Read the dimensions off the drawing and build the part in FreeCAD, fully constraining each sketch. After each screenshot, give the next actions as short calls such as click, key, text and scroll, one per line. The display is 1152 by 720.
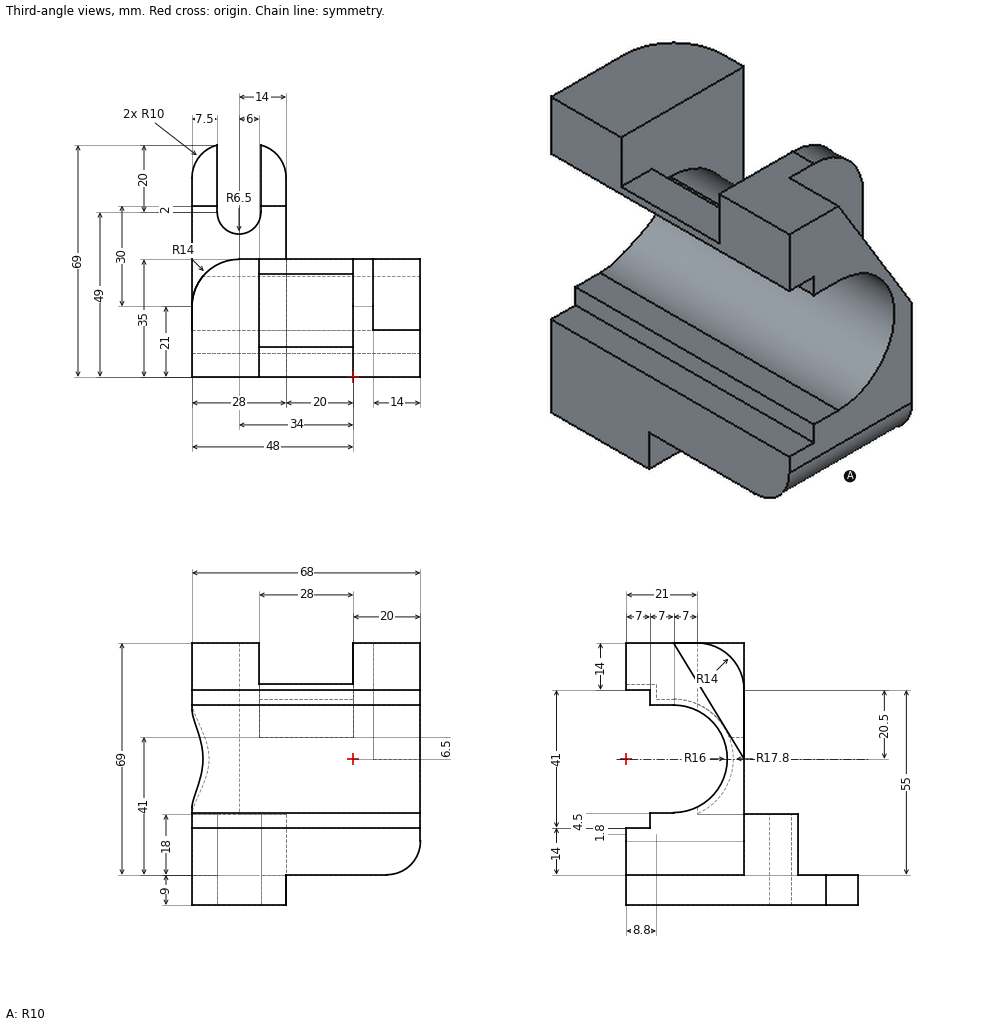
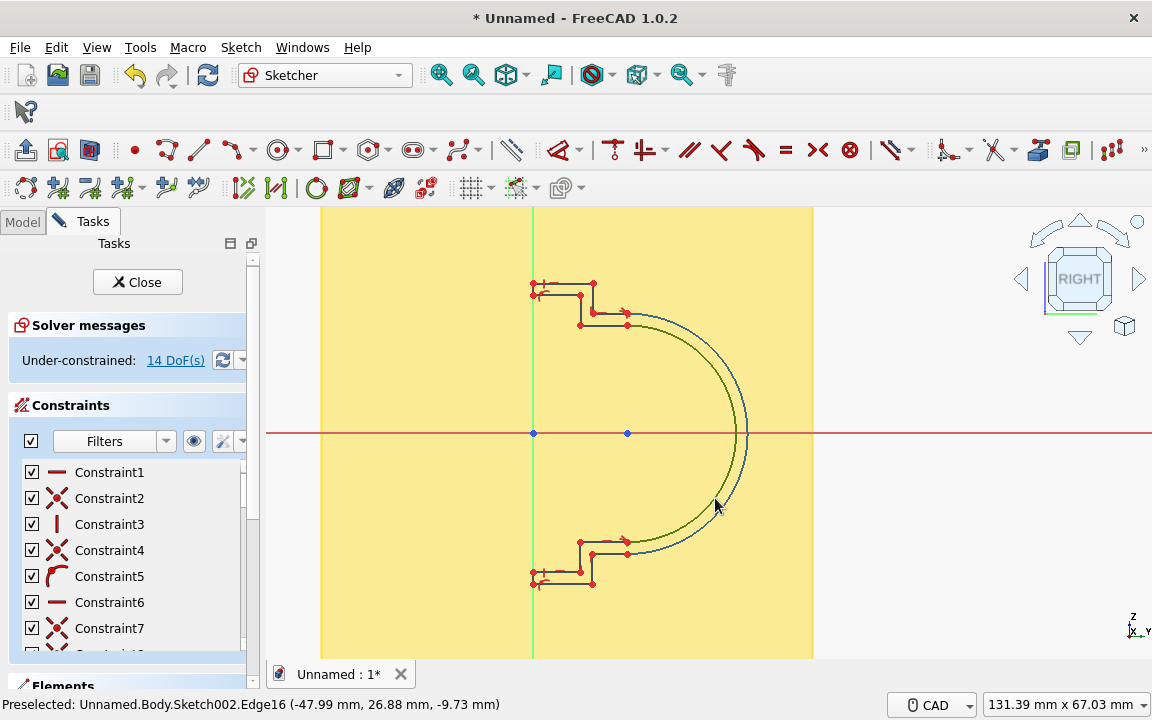
click(614, 150)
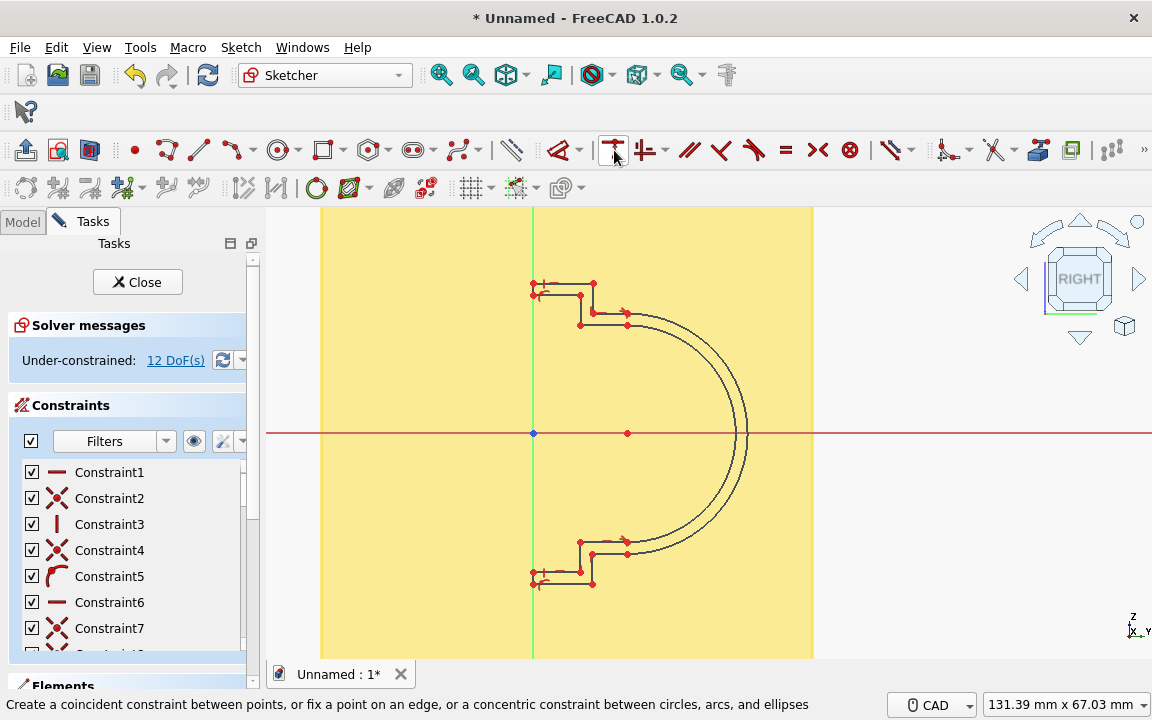
click(627, 434)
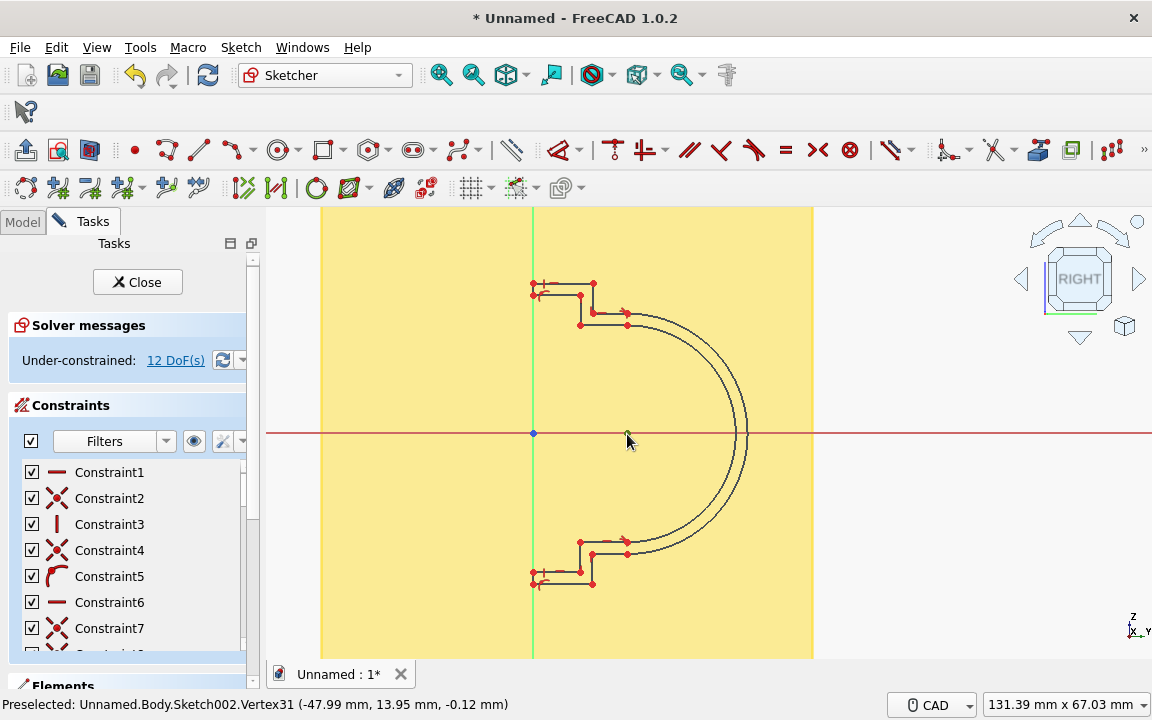
click(344, 433)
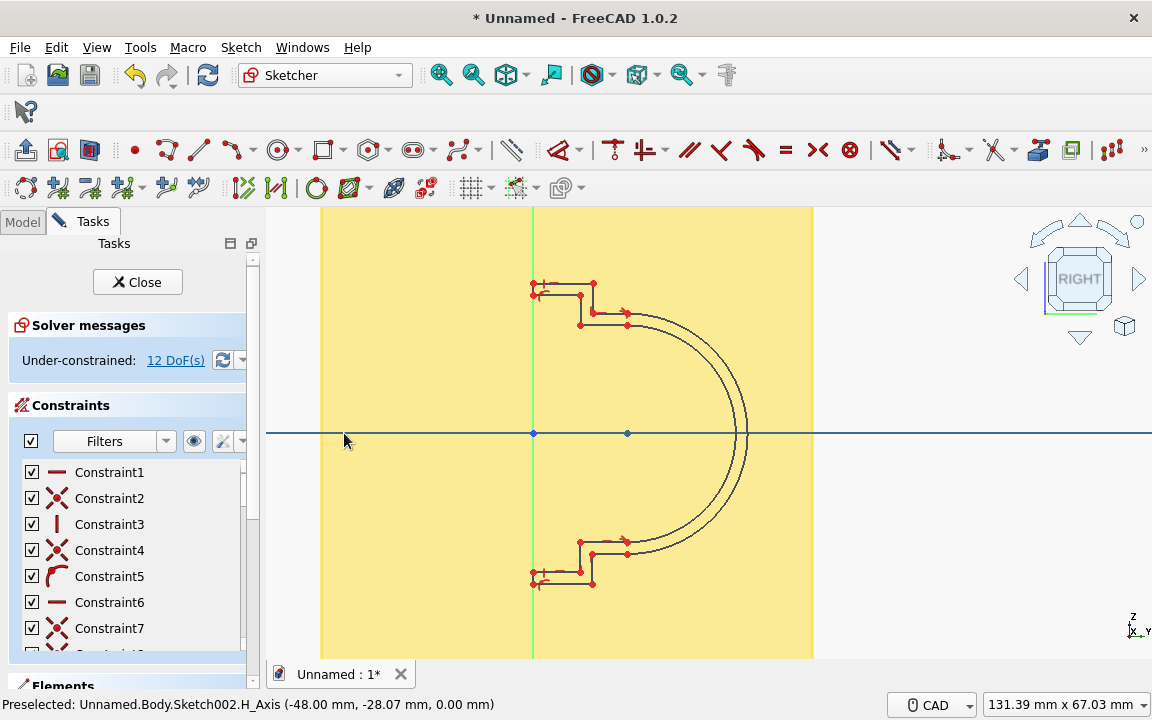
click(614, 150)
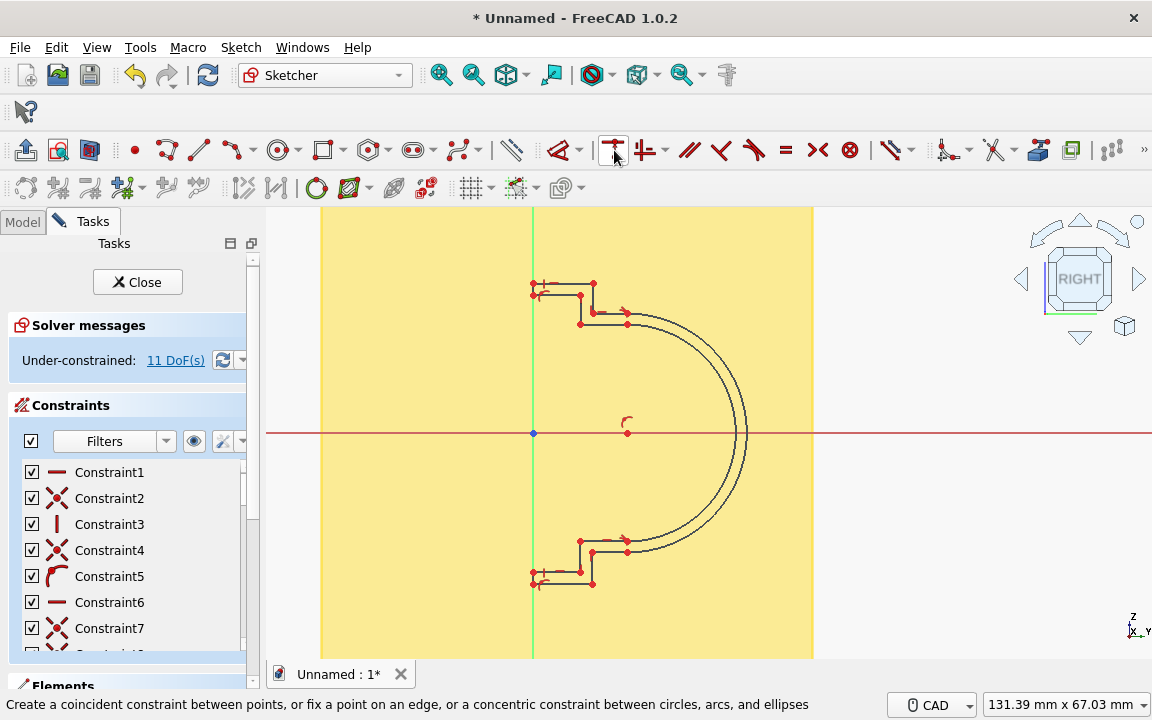
click(592, 584)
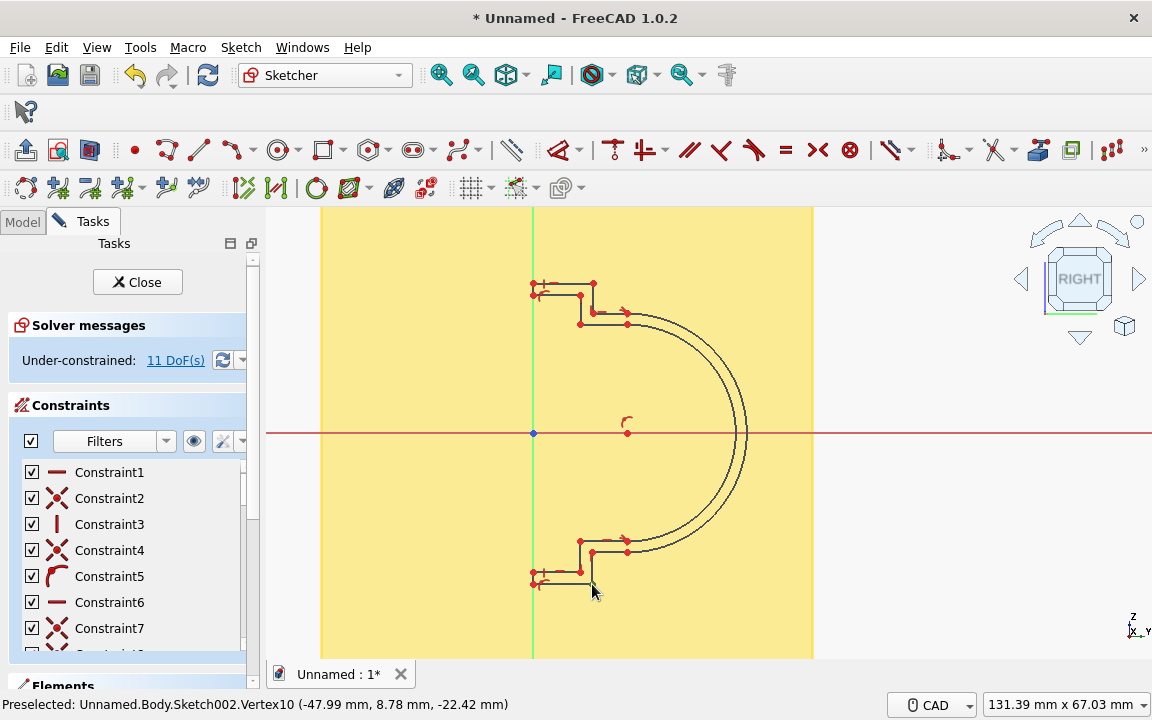
click(593, 284)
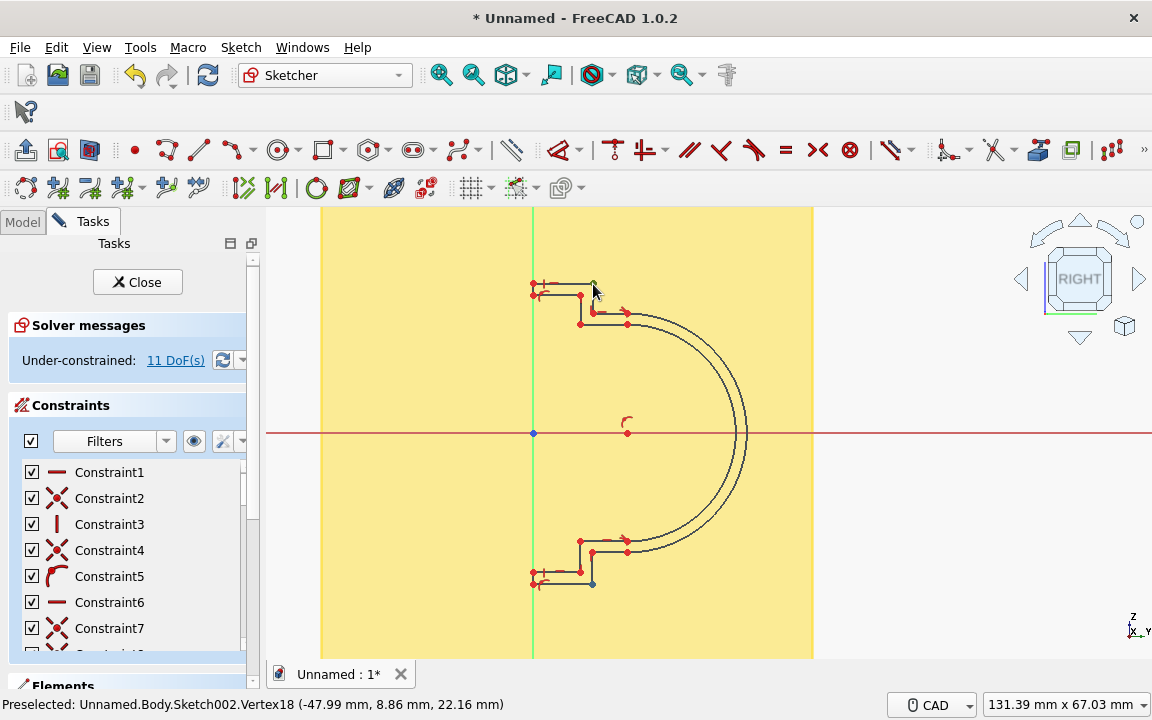
click(344, 433)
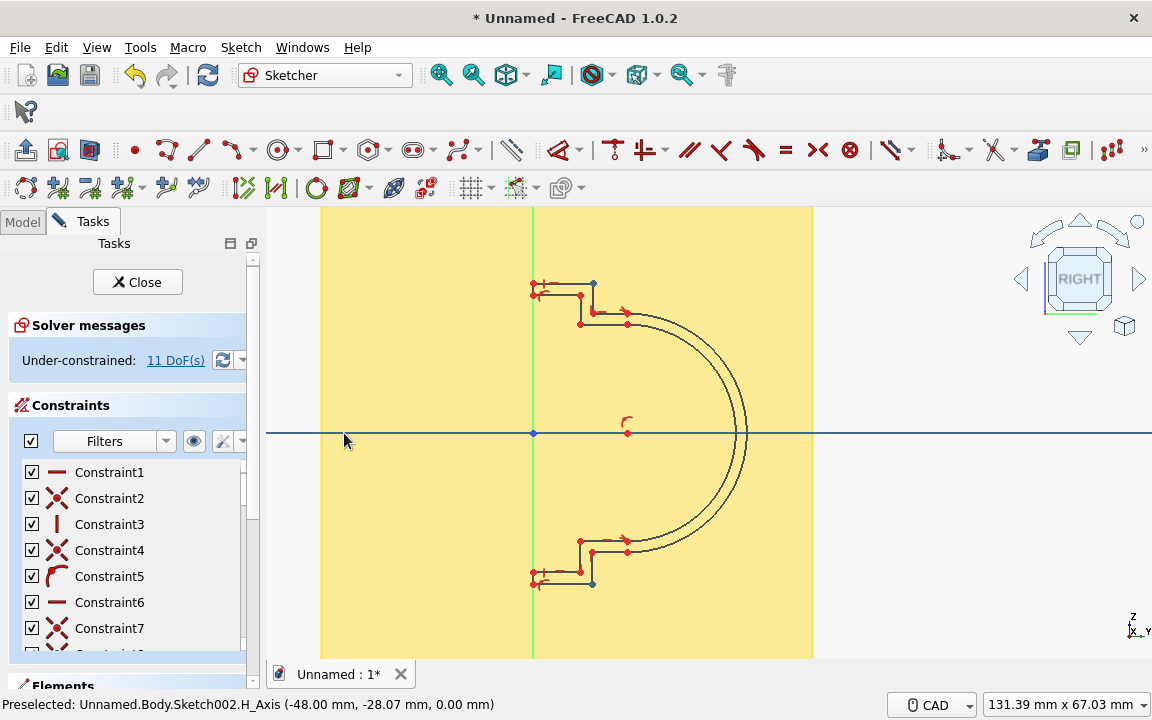
click(818, 150)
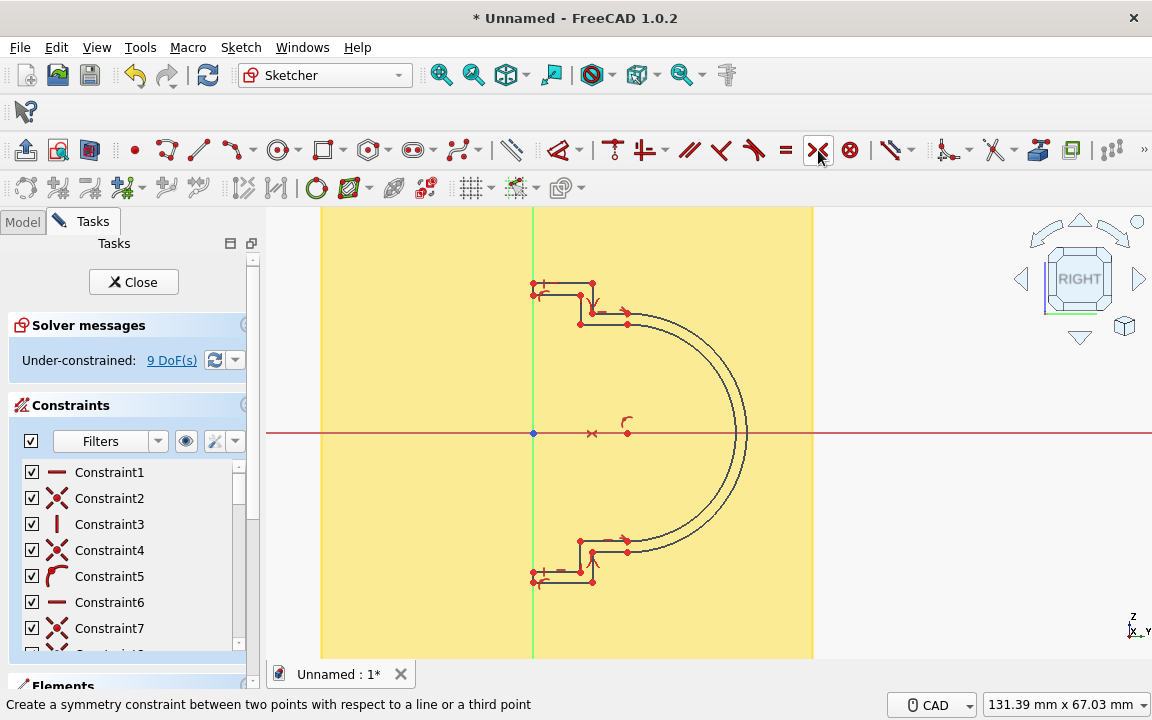
click(580, 572)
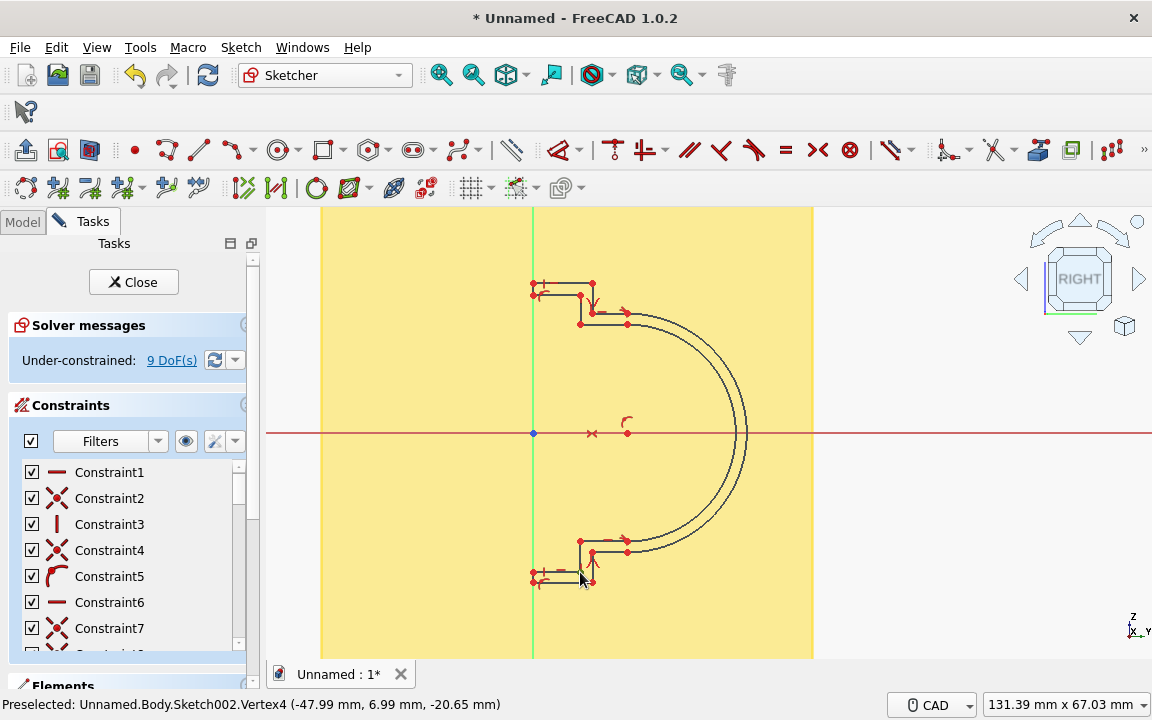
click(581, 295)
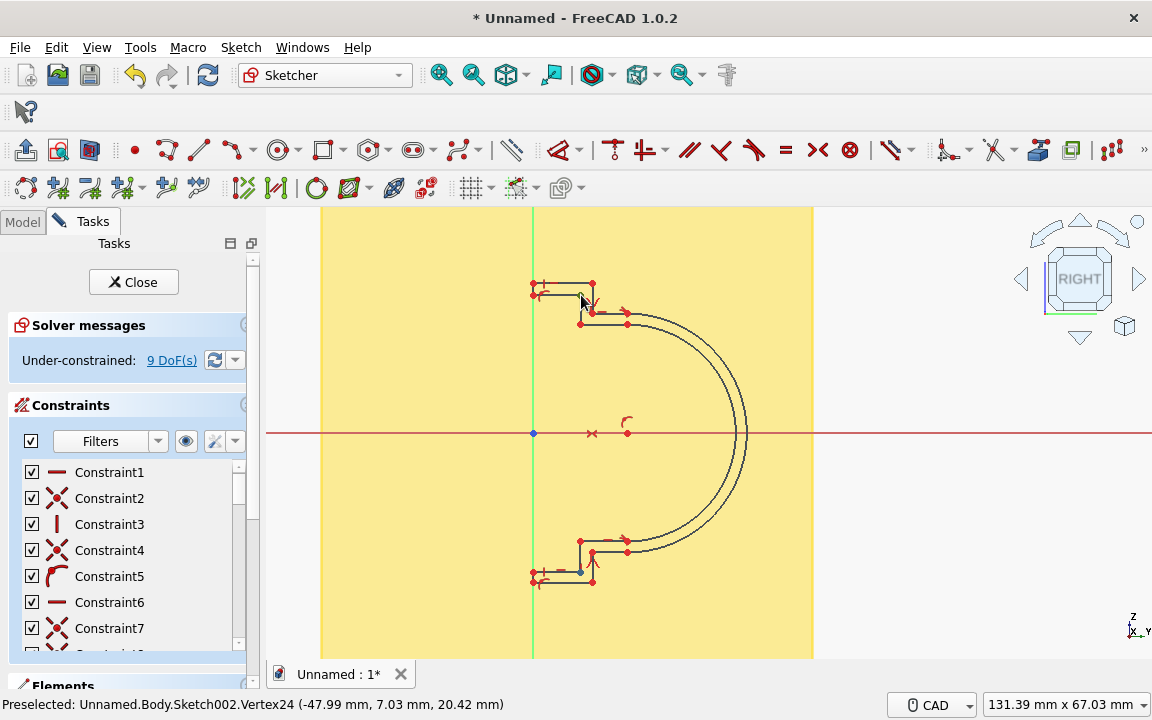
click(344, 433)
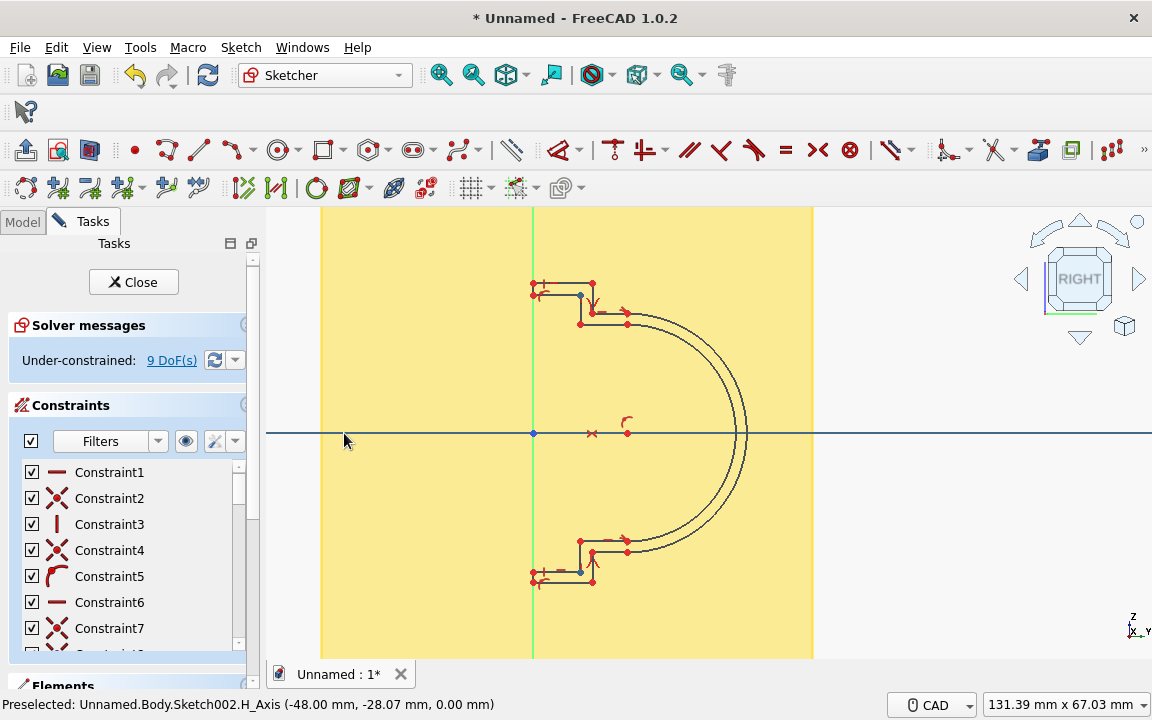
click(818, 150)